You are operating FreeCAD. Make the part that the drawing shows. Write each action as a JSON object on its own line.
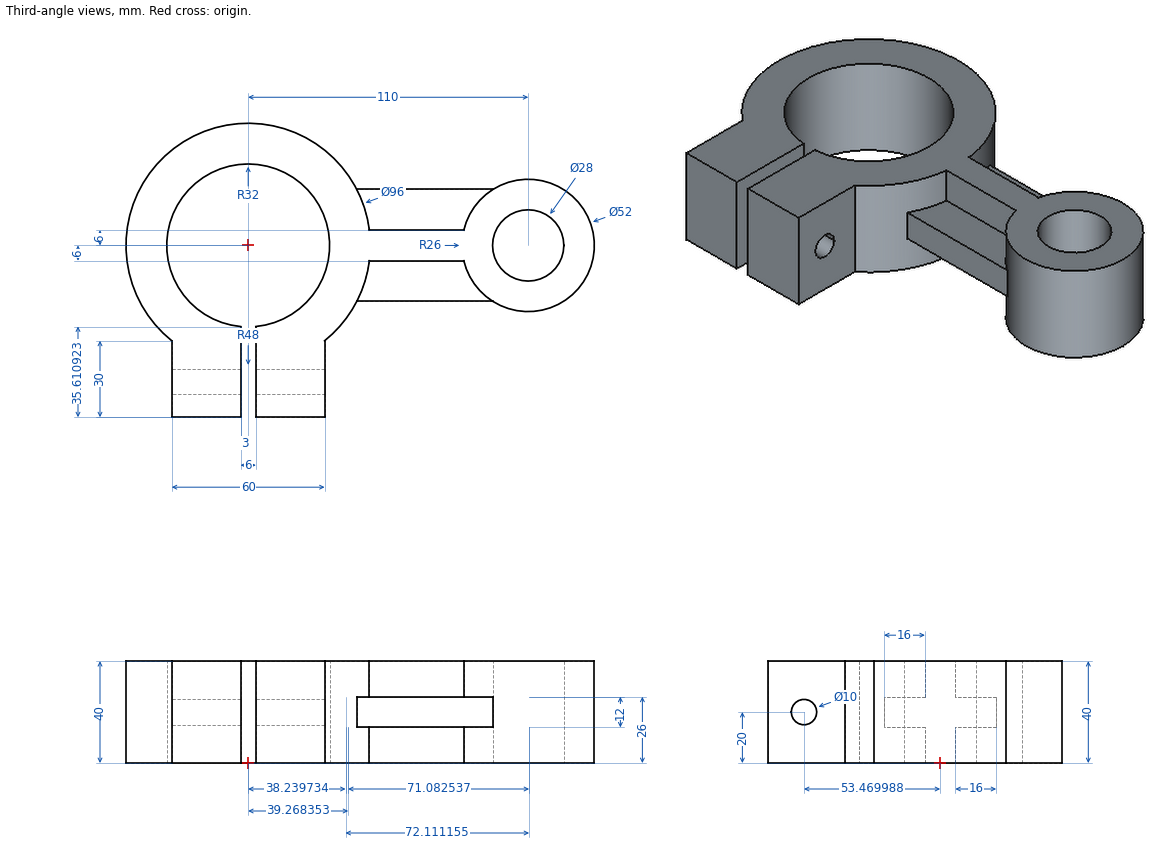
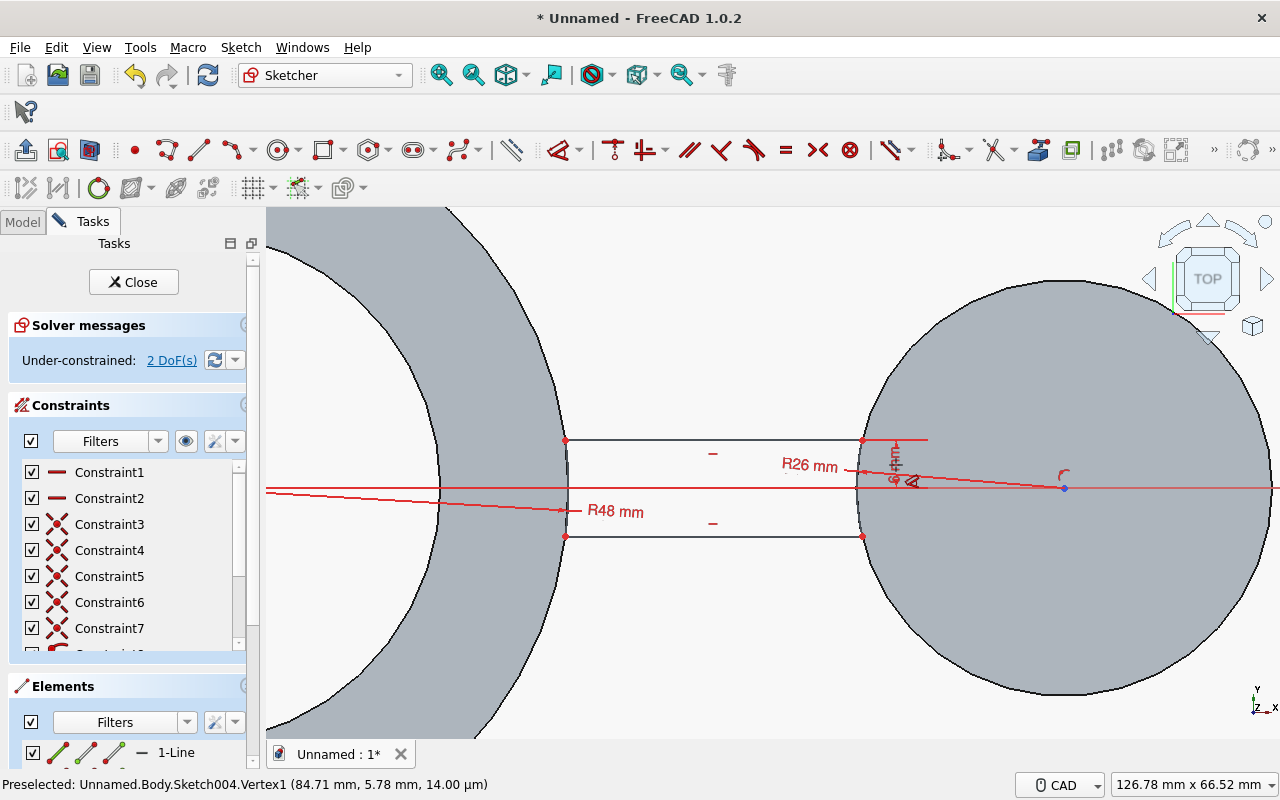
{"action": "left_click", "coordinate": [565, 537]}
{"action": "left_click", "coordinate": [695, 513]}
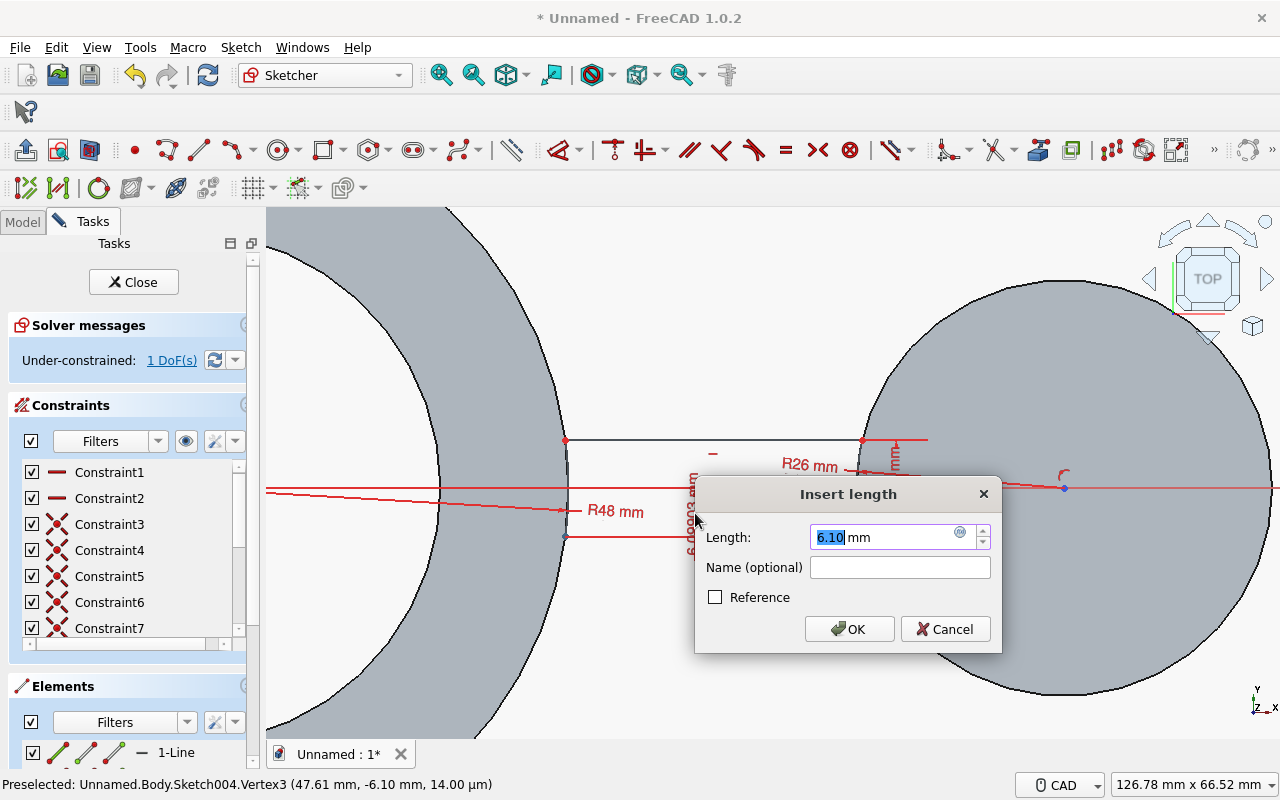
{"action": "type", "text": "6"}
{"action": "key", "text": "Return"}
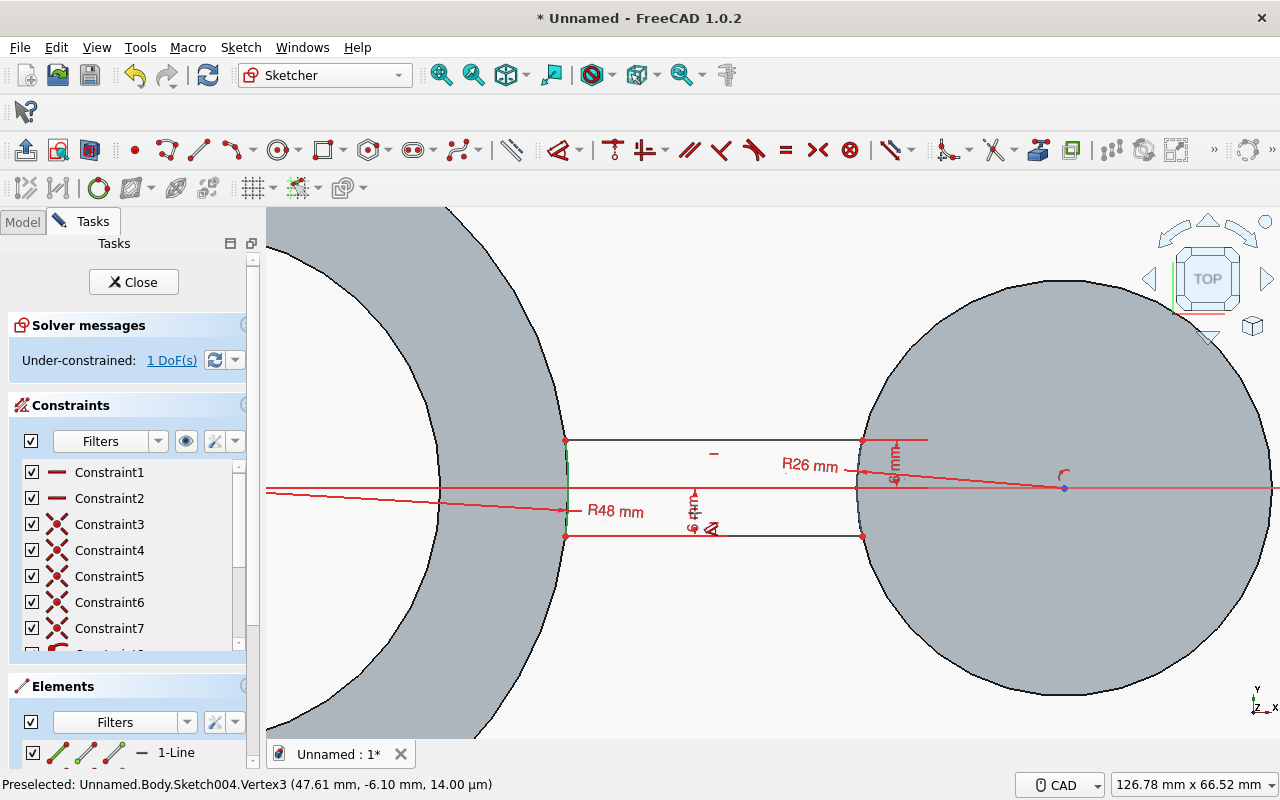
{"action": "left_click", "coordinate": [1065, 488]}
{"action": "left_click", "coordinate": [502, 522]}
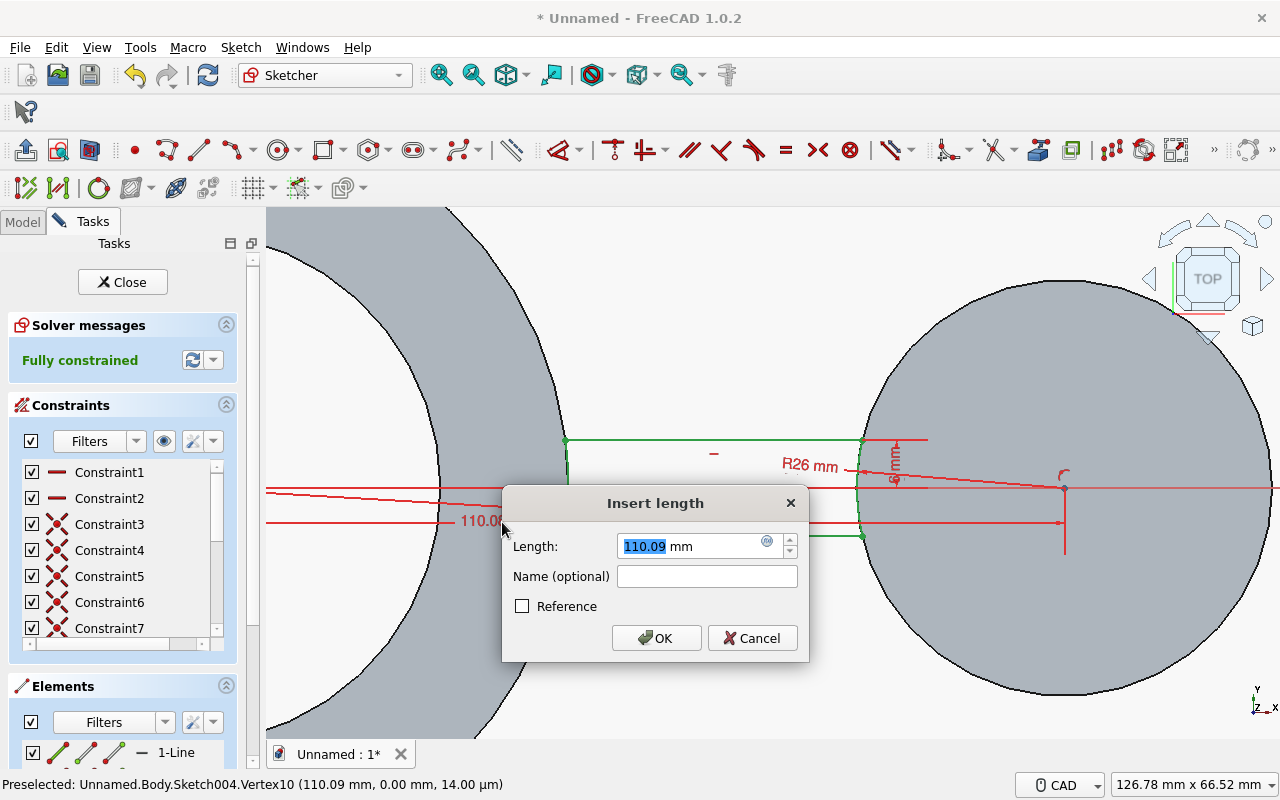
{"action": "type", "text": "110"}
{"action": "key", "text": "Return"}
{"action": "key", "text": "Escape"}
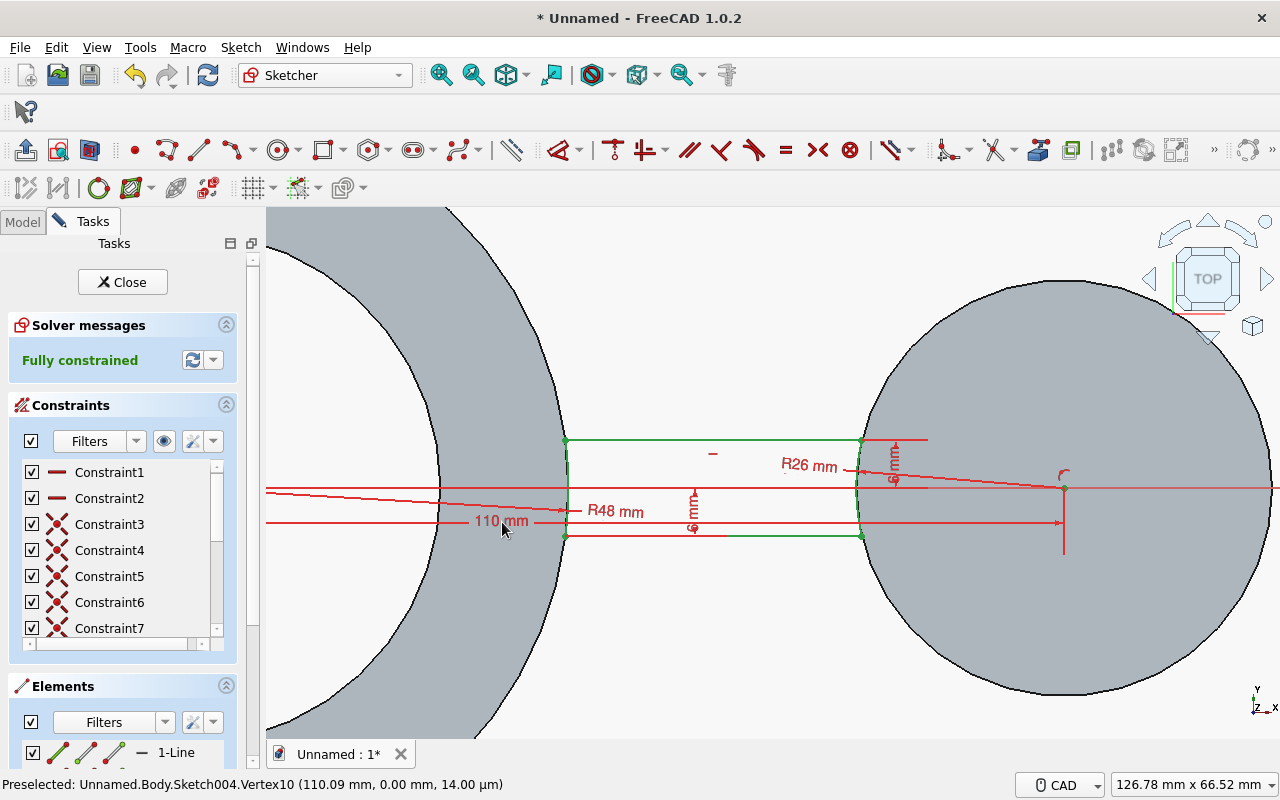
{"action": "left_click", "coordinate": [123, 282]}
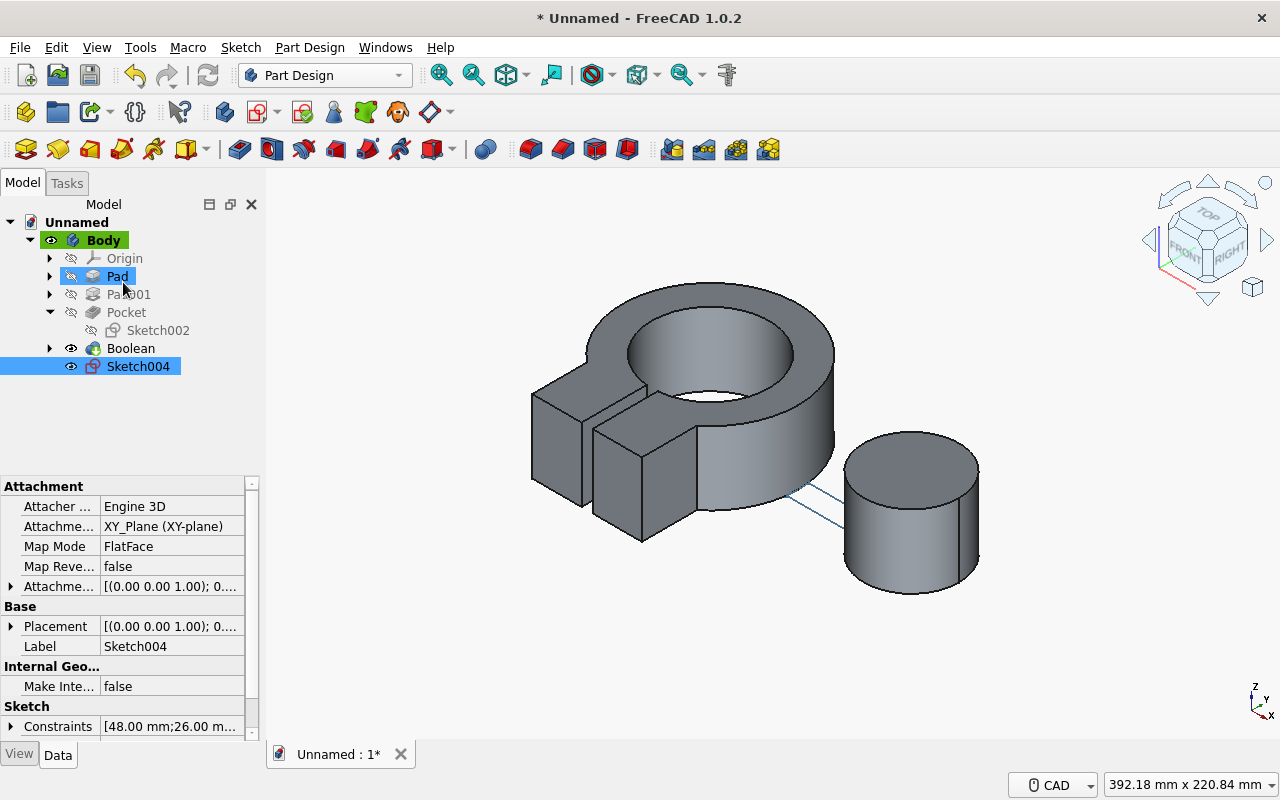
{"action": "left_click", "coordinate": [26, 150]}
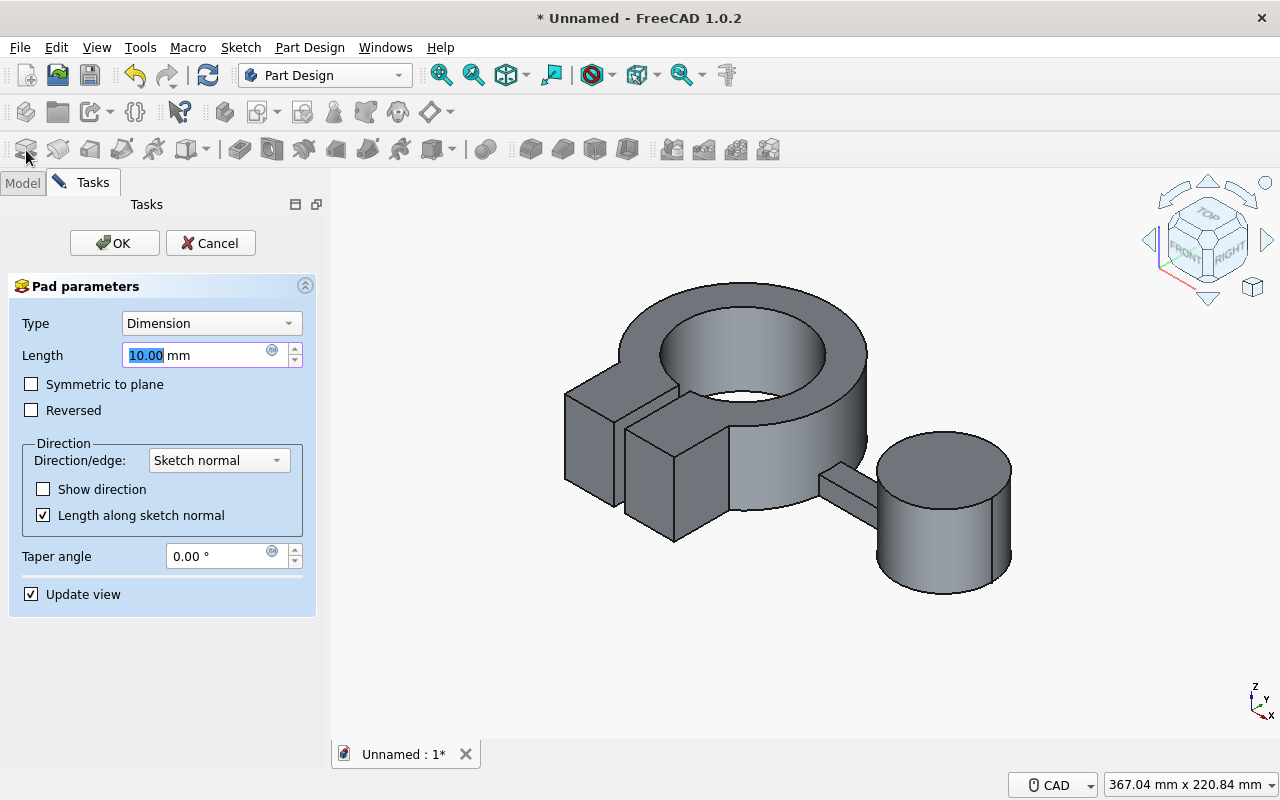
{"action": "type", "text": "40"}
{"action": "key", "text": "Tab"}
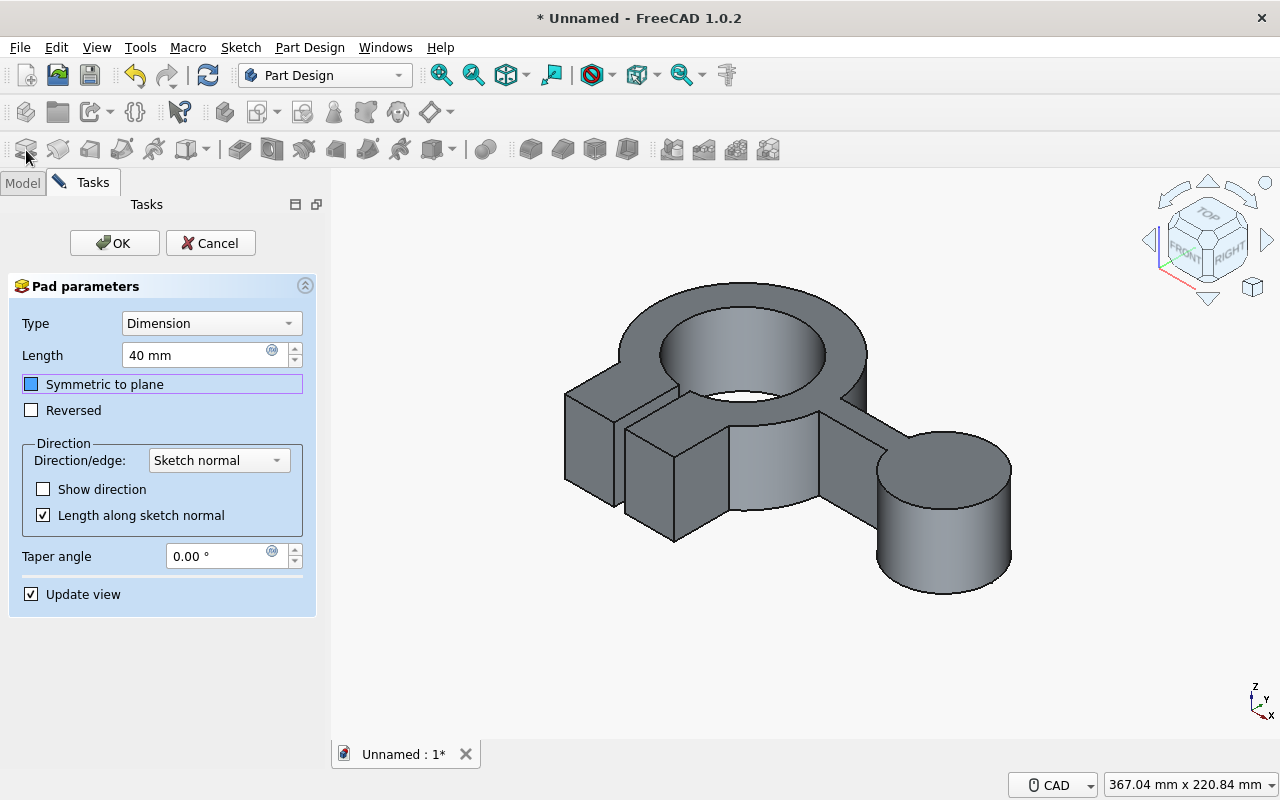
{"action": "left_click", "coordinate": [115, 243]}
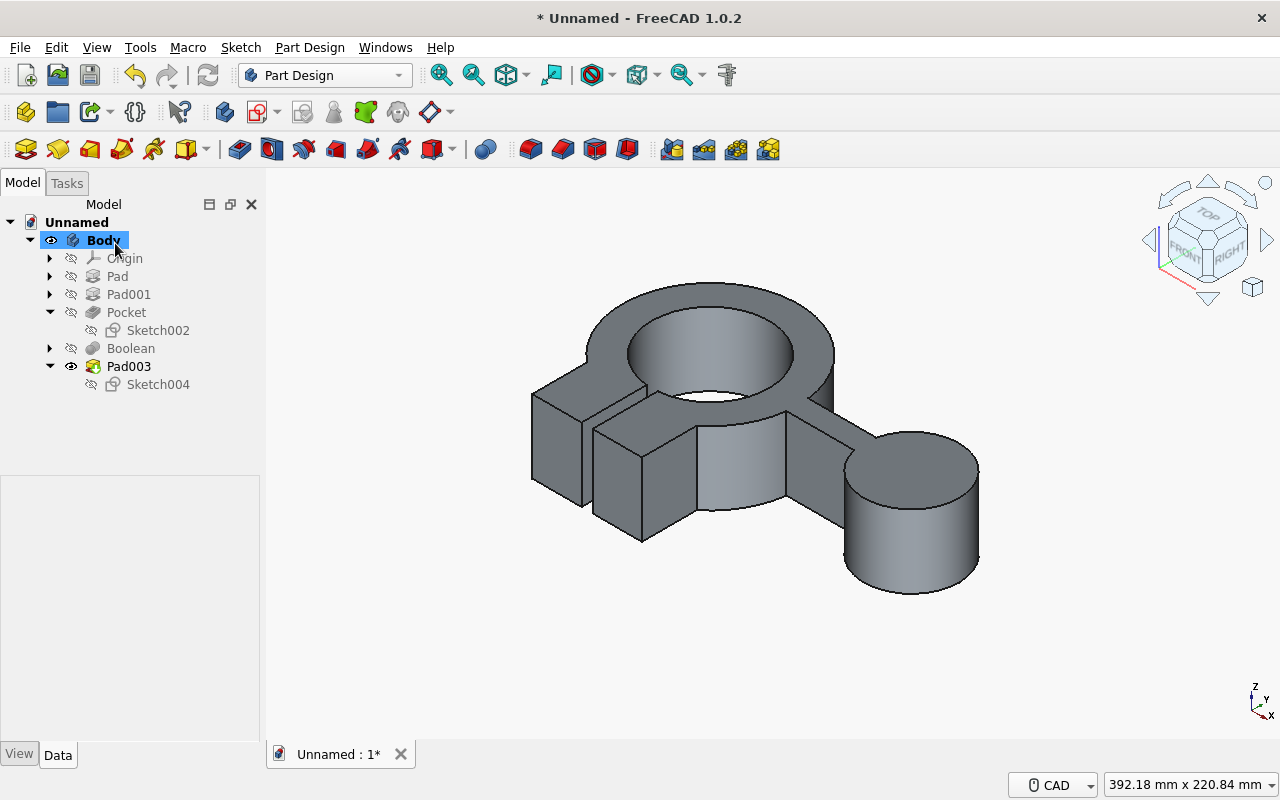
{"action": "key", "text": "4"}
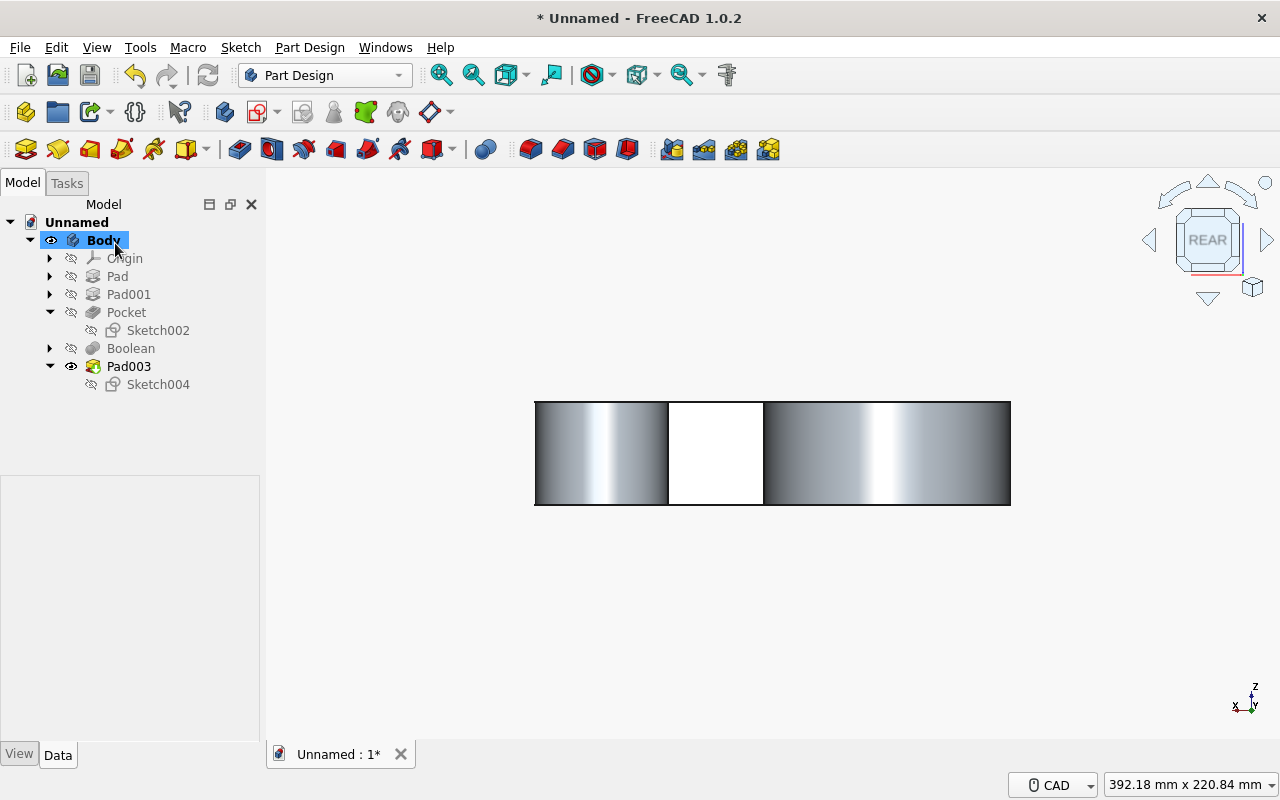
{"action": "left_click", "coordinate": [716, 453]}